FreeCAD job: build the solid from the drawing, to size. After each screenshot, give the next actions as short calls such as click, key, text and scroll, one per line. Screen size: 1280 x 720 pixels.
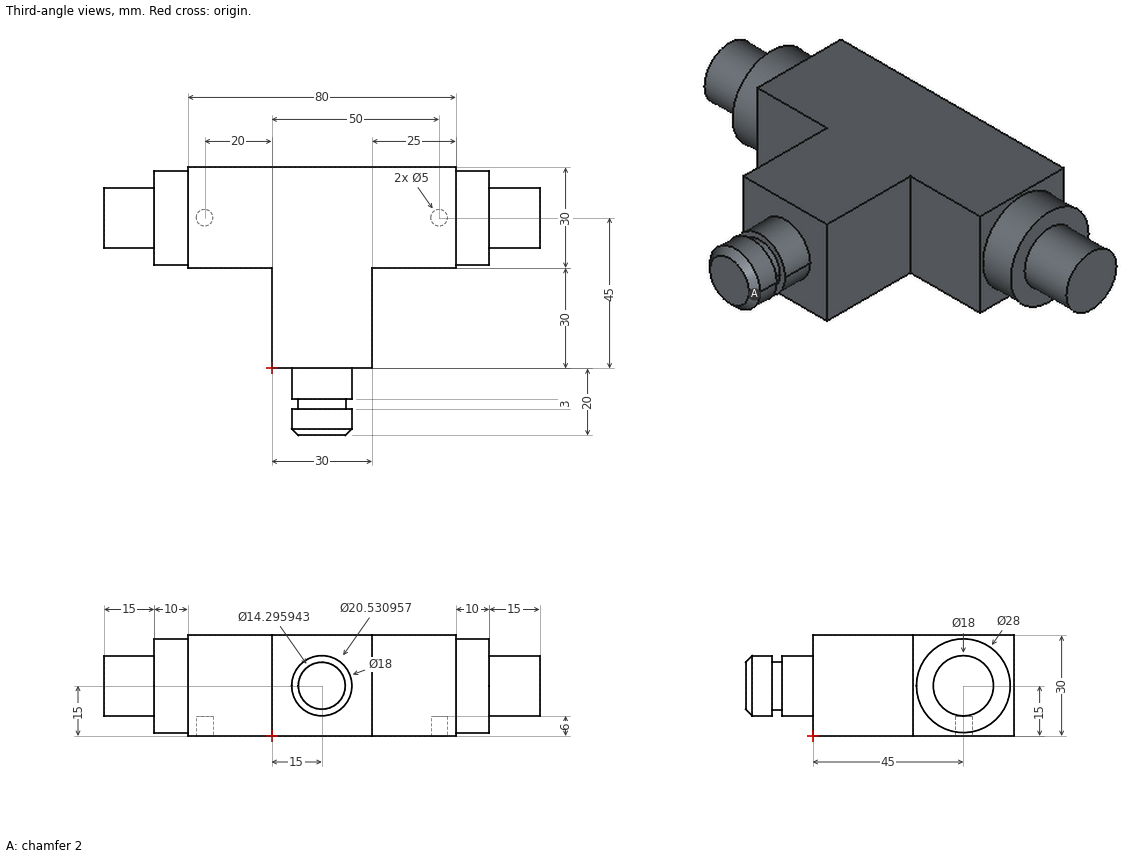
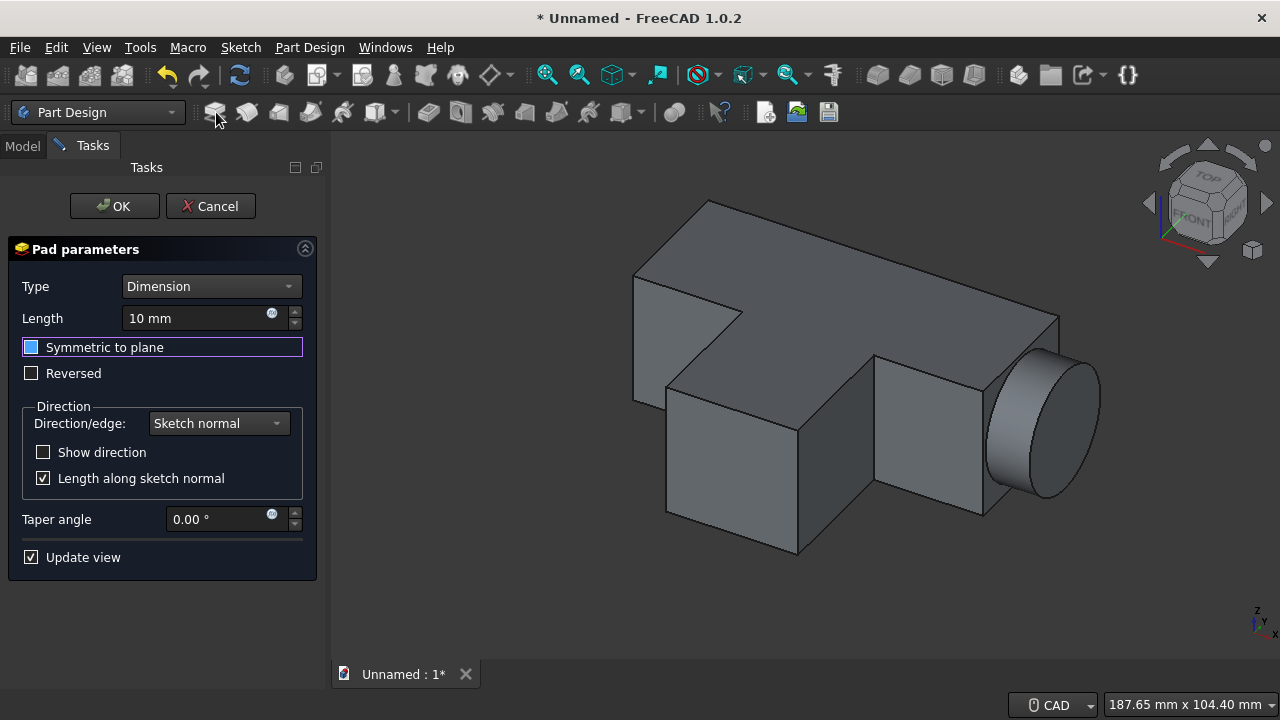
click(115, 206)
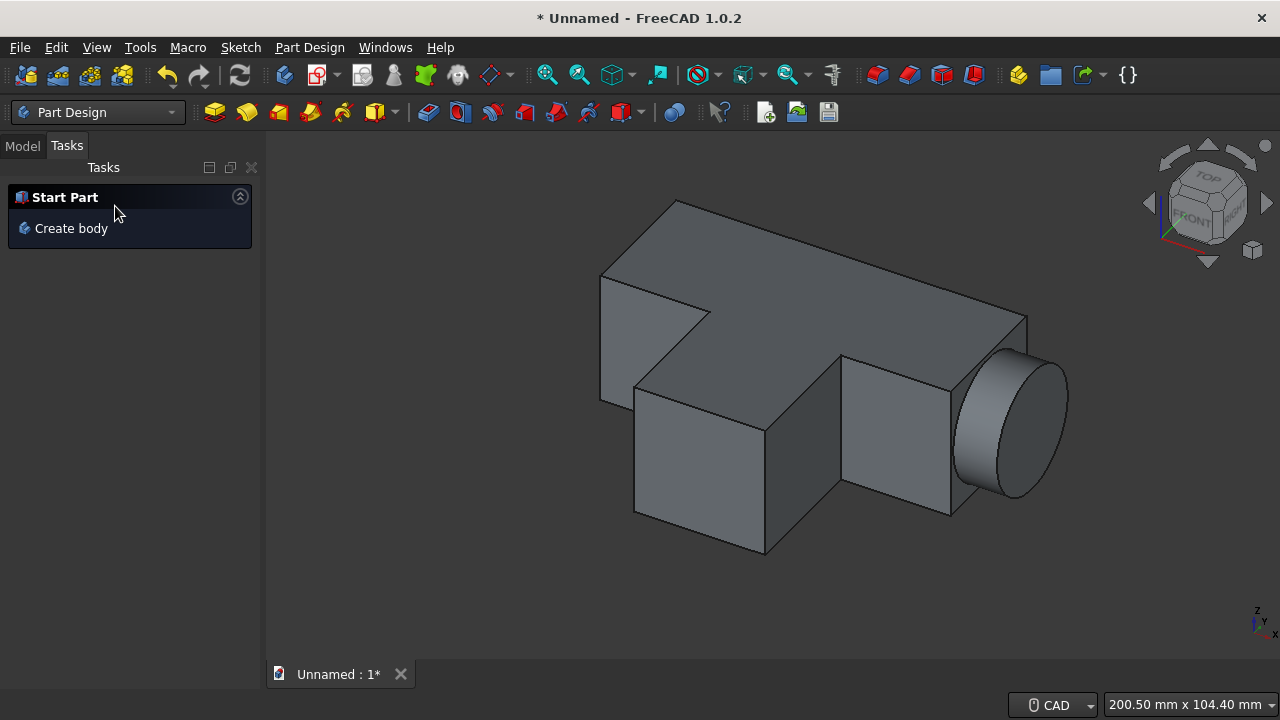
click(1032, 430)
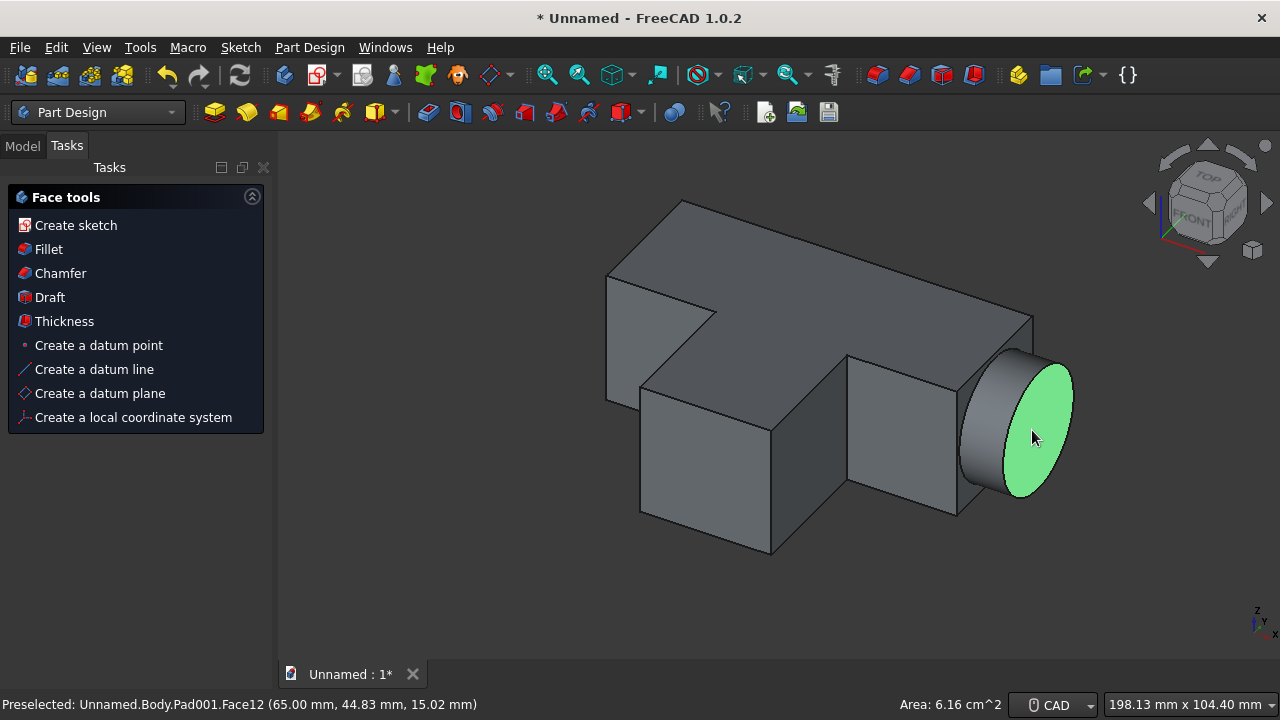
click(318, 76)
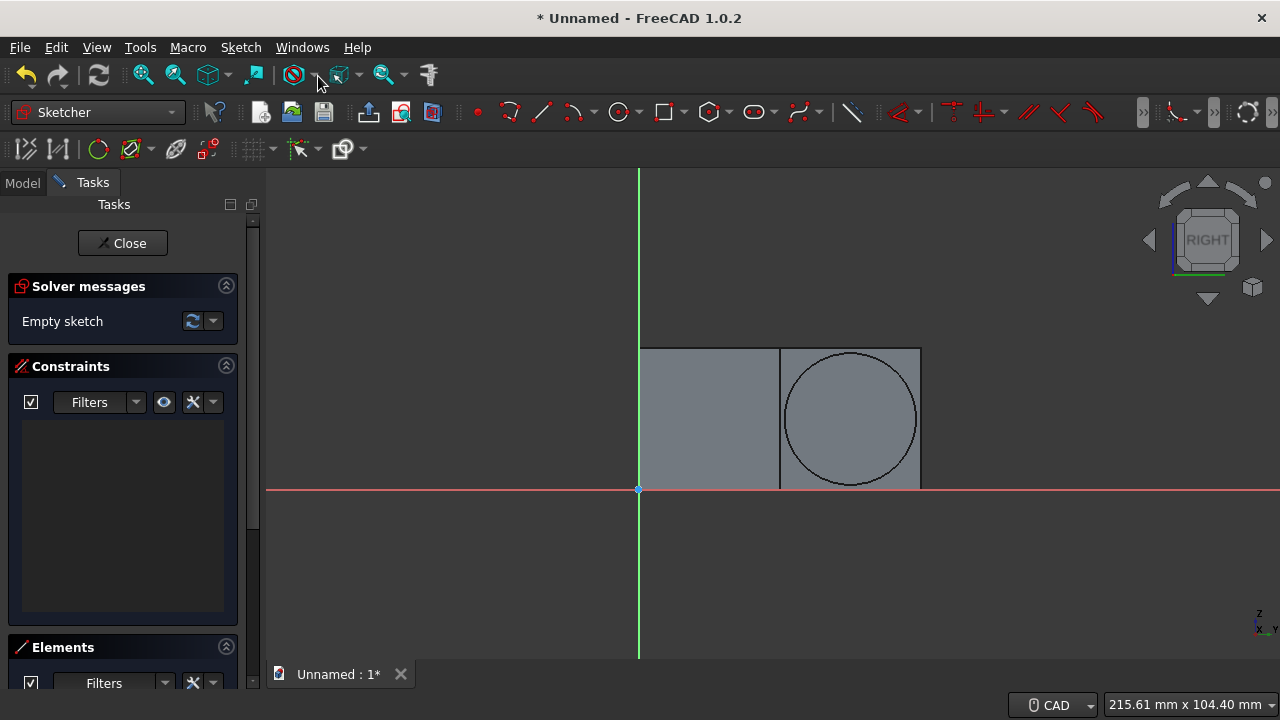
scroll(913, 421, up, 6)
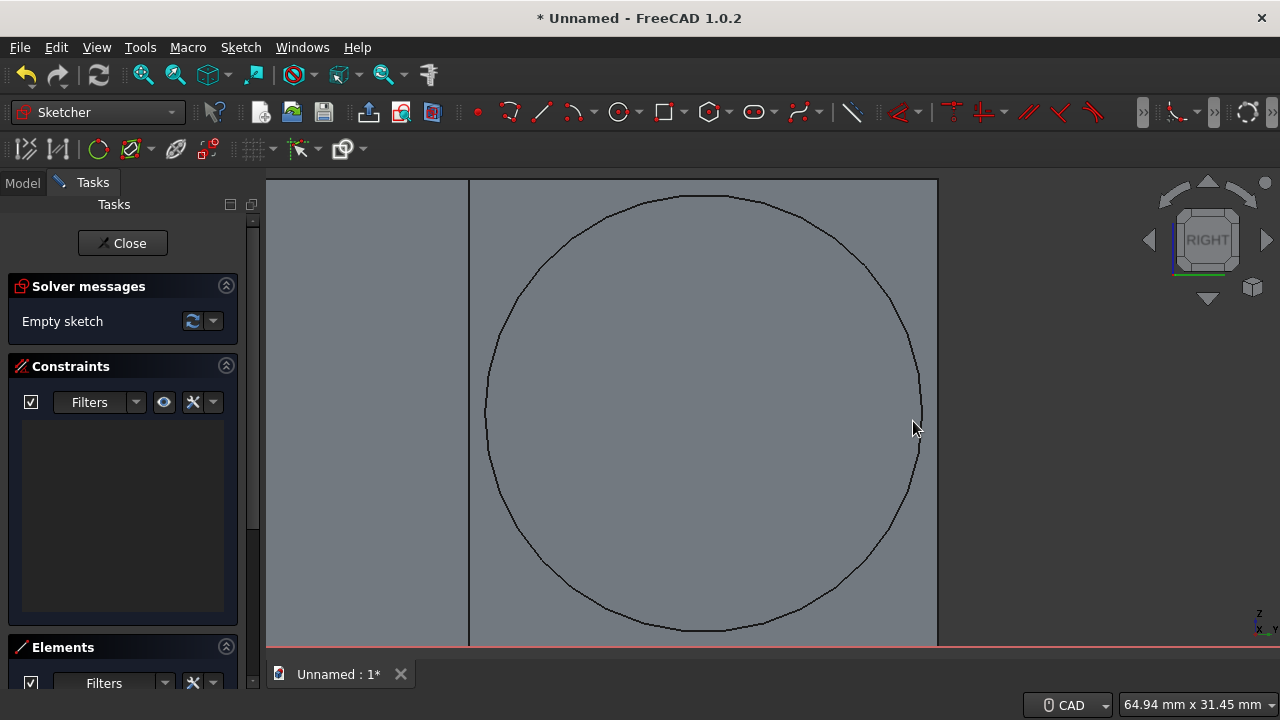
key(g)
key(c)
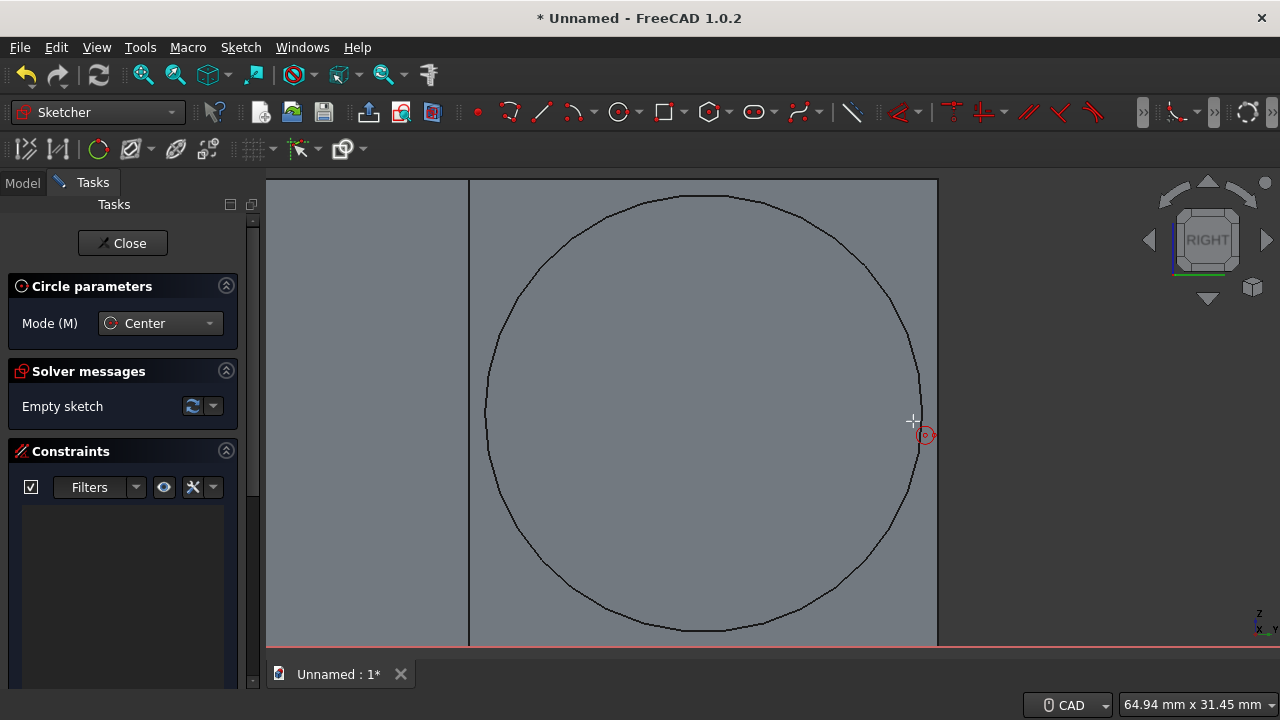
click(704, 413)
move(803, 314)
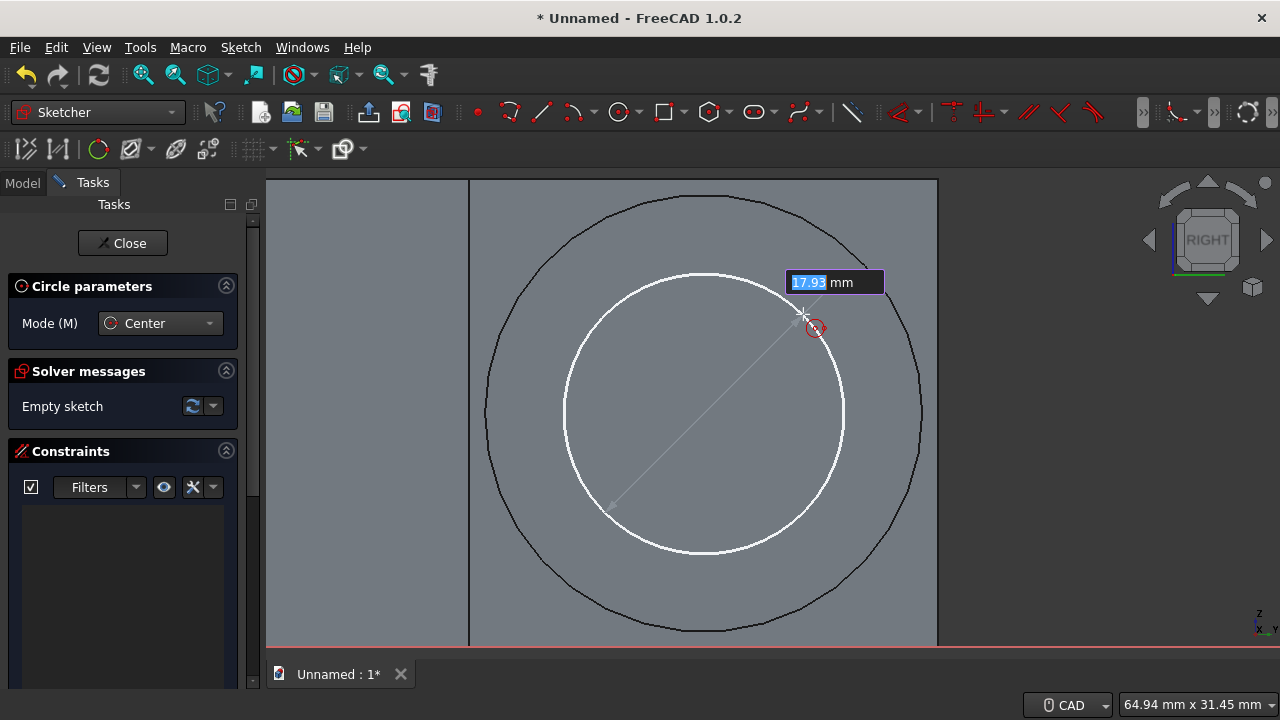
text(18)
key(Return)
key(Escape)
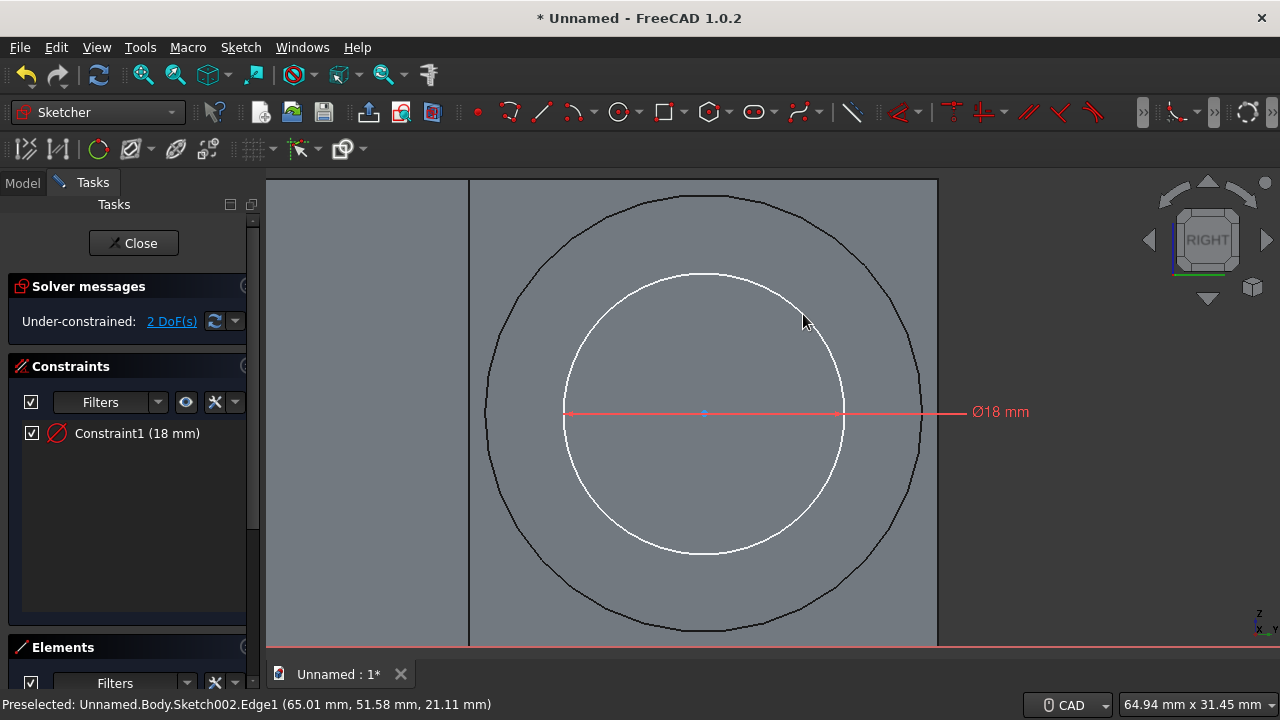
key(d)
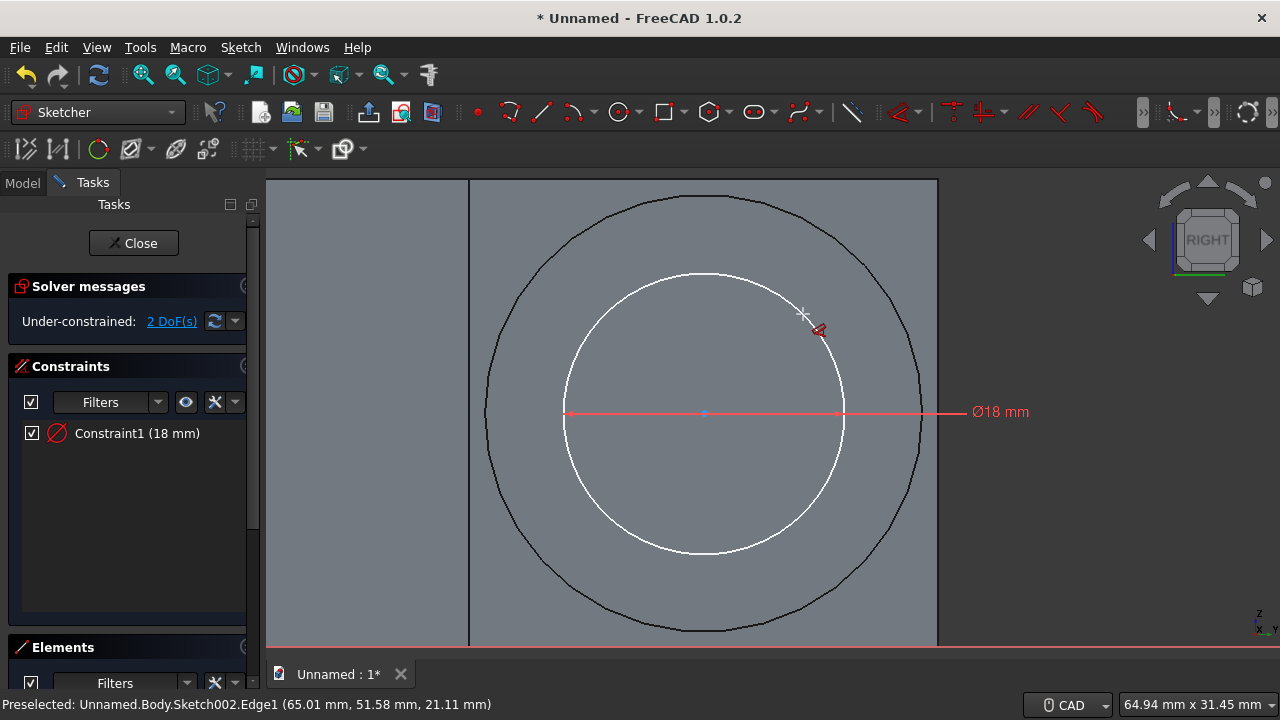
click(704, 414)
click(499, 380)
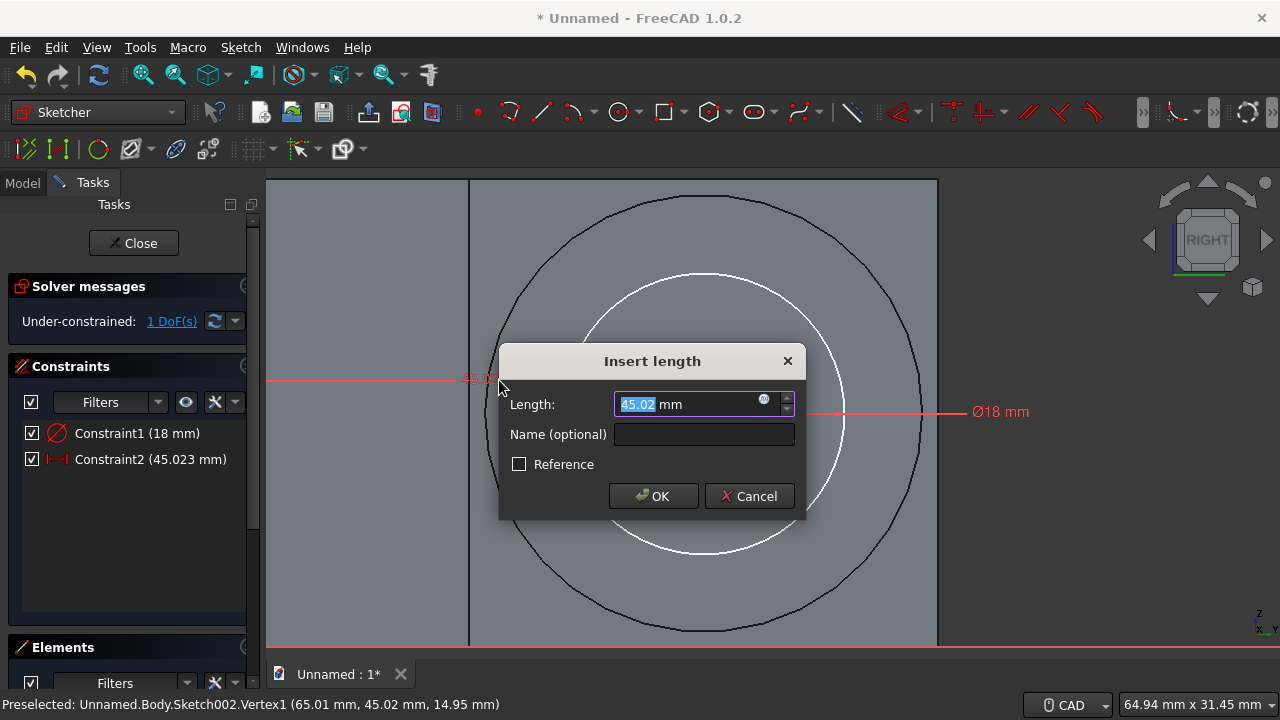
text(45)
key(Return)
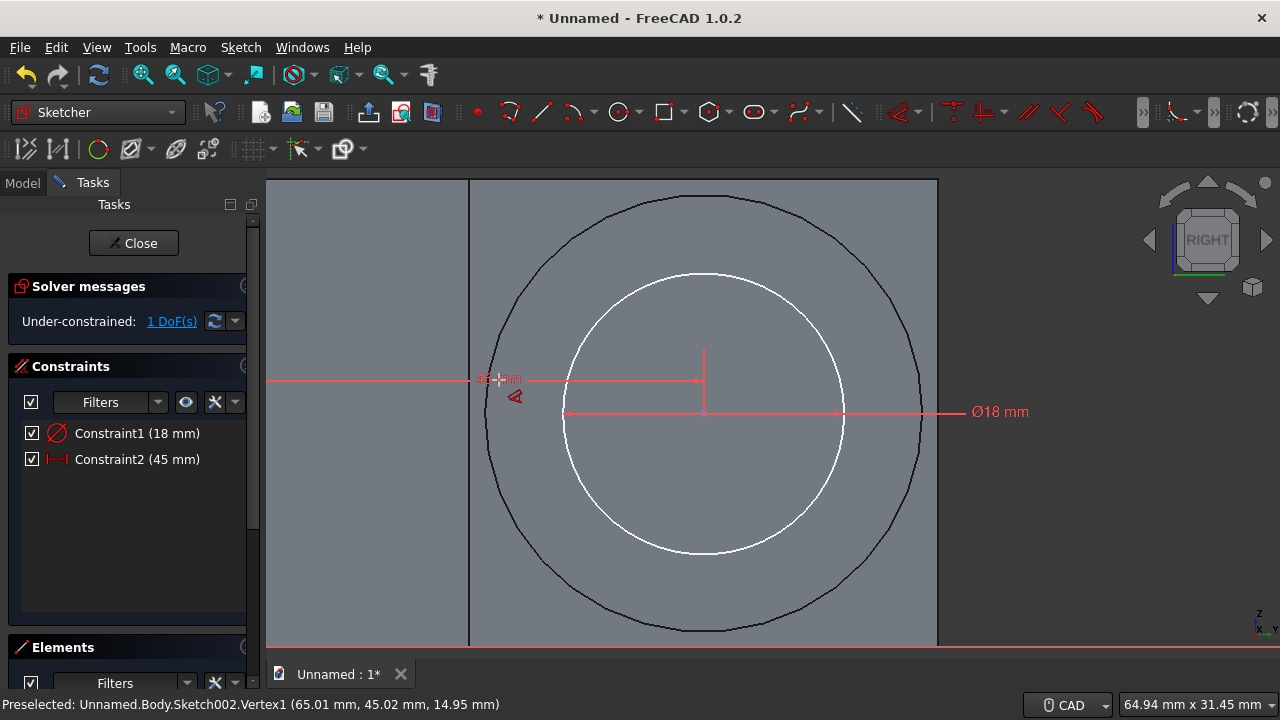
click(704, 414)
click(738, 522)